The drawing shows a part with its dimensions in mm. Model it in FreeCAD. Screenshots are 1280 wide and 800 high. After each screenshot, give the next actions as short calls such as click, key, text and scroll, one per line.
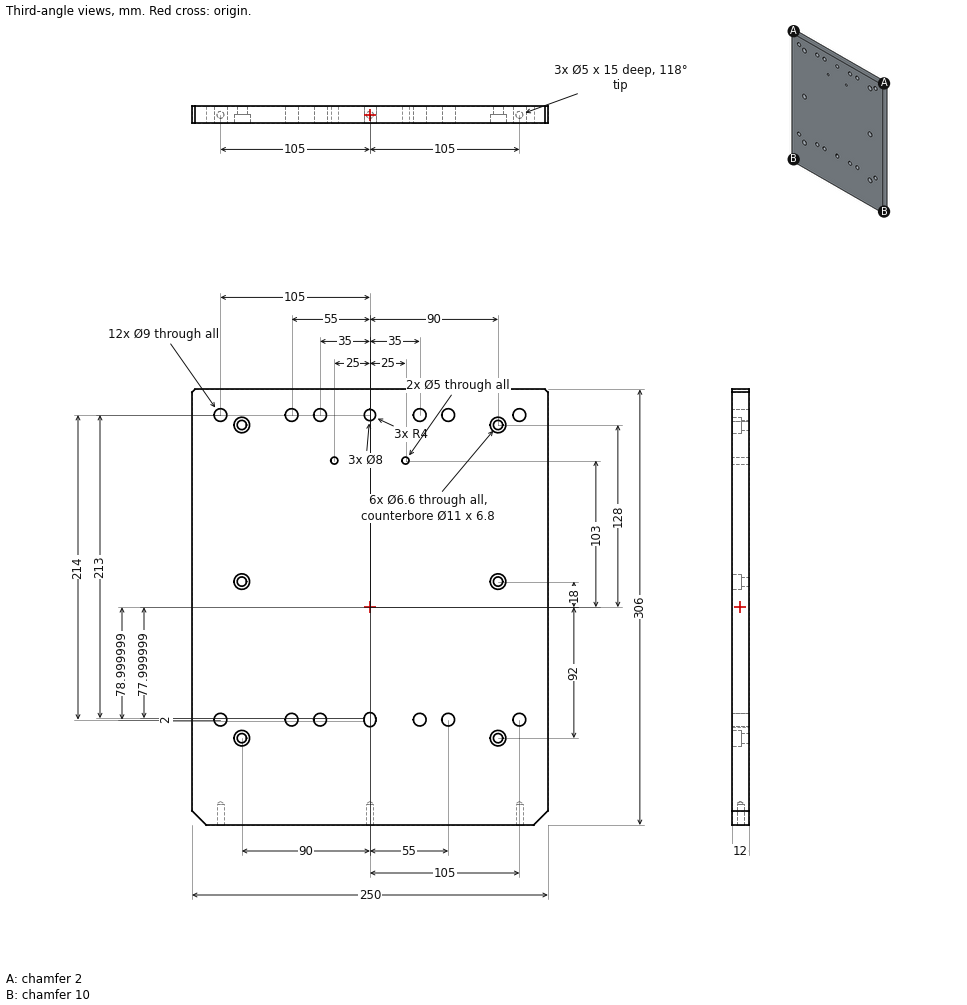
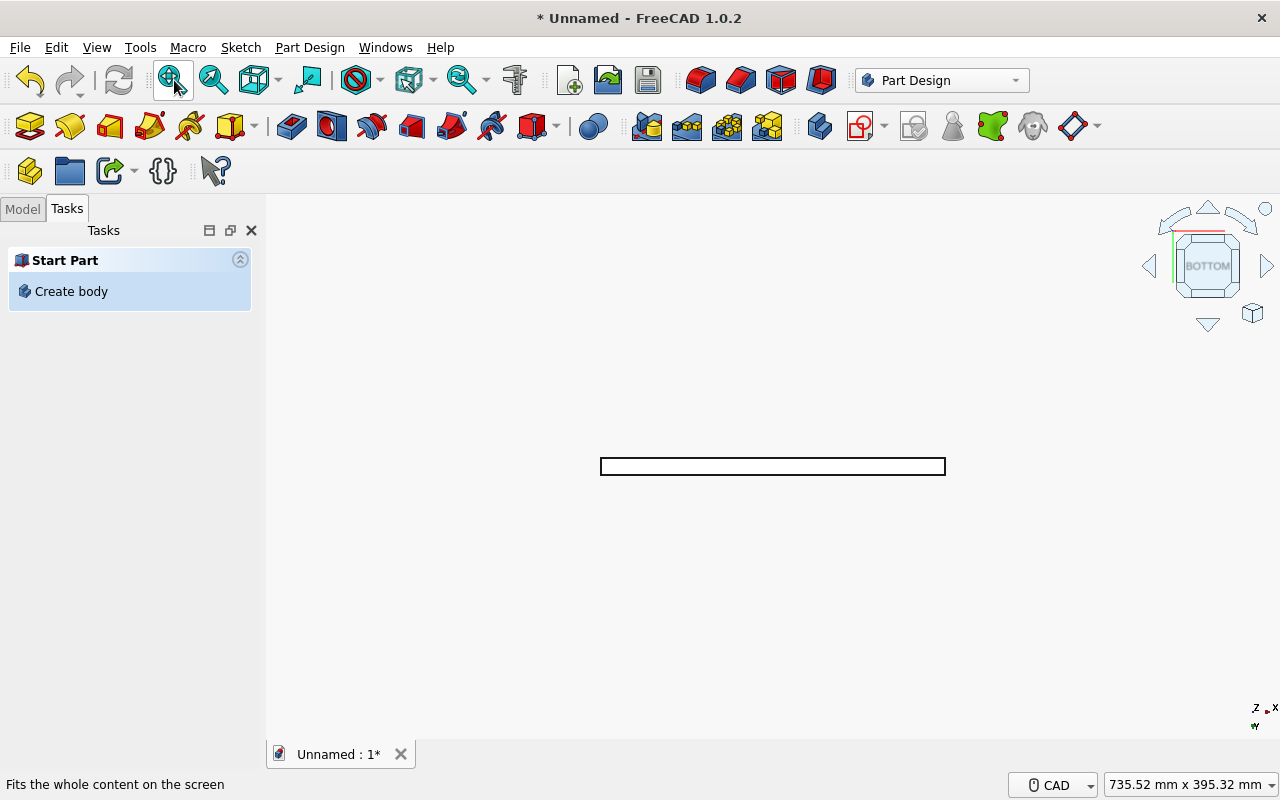
key(1)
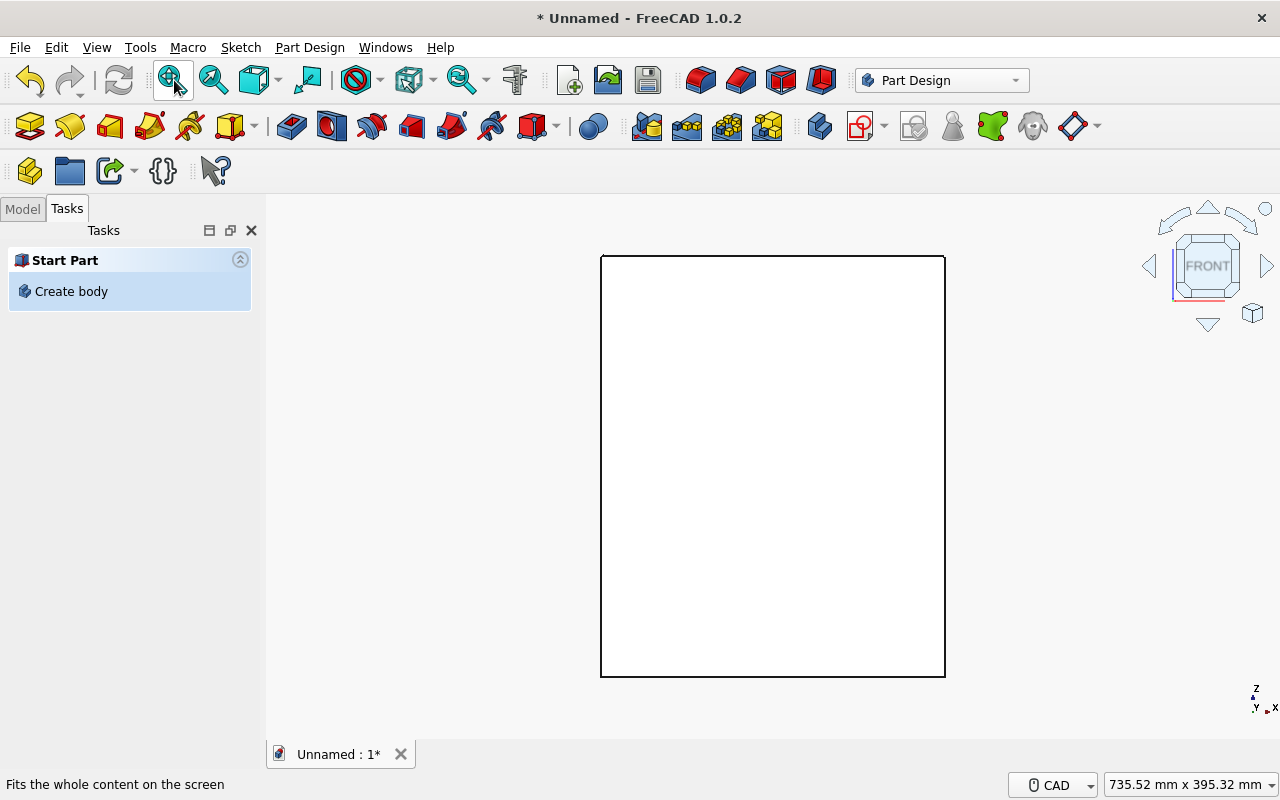
key(3)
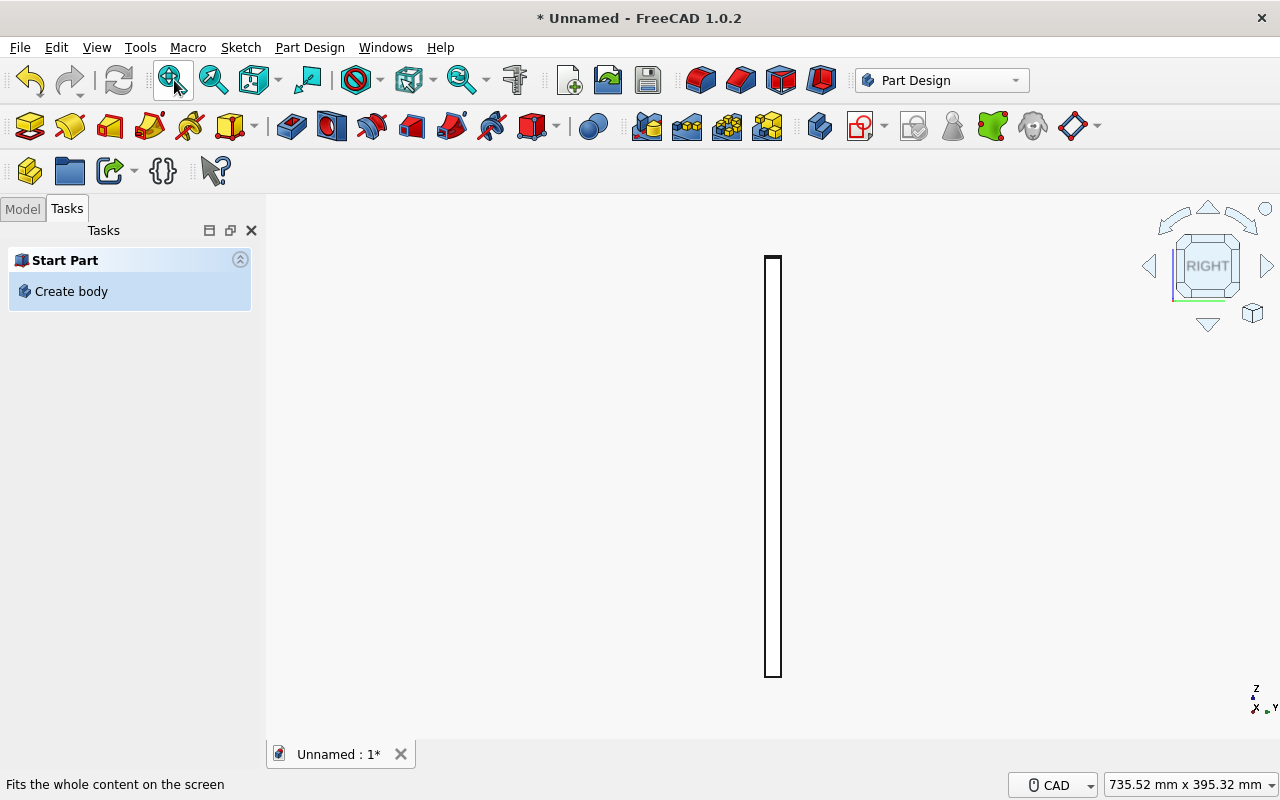
click(23, 208)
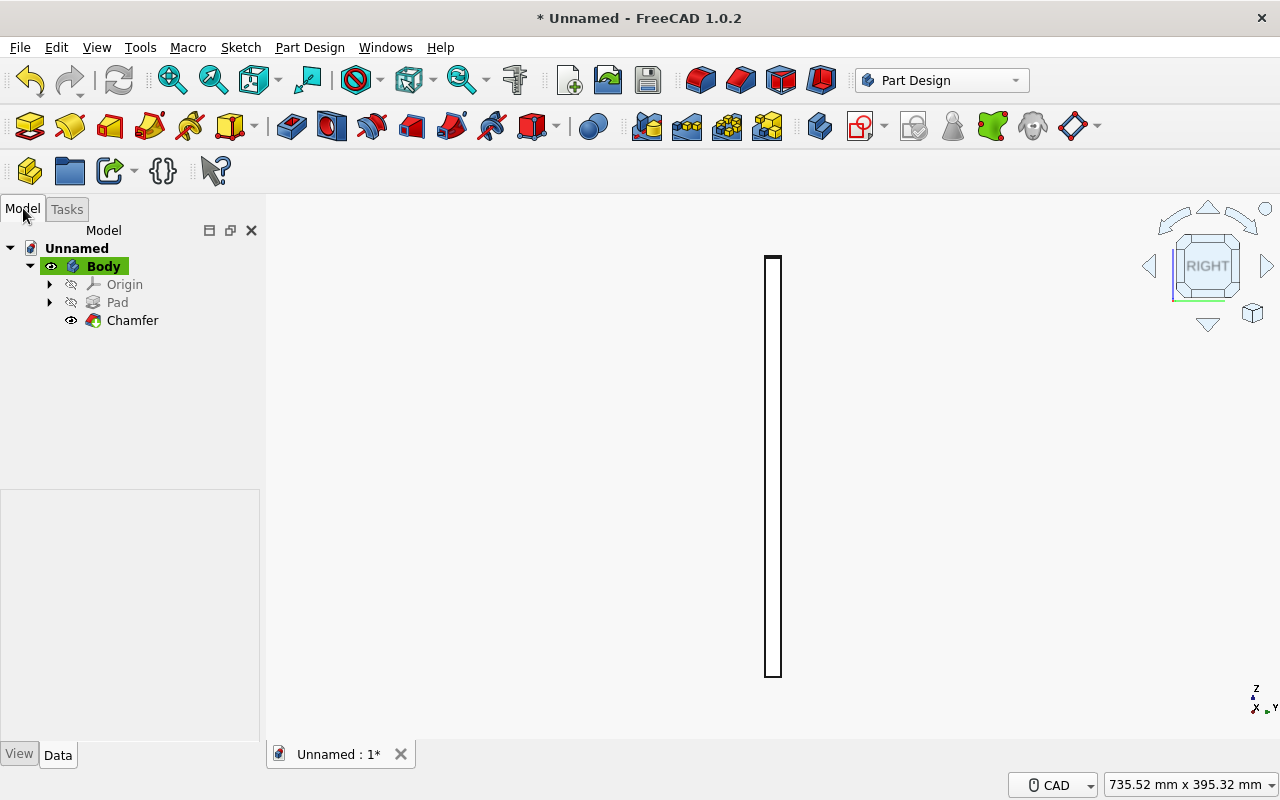
click(50, 284)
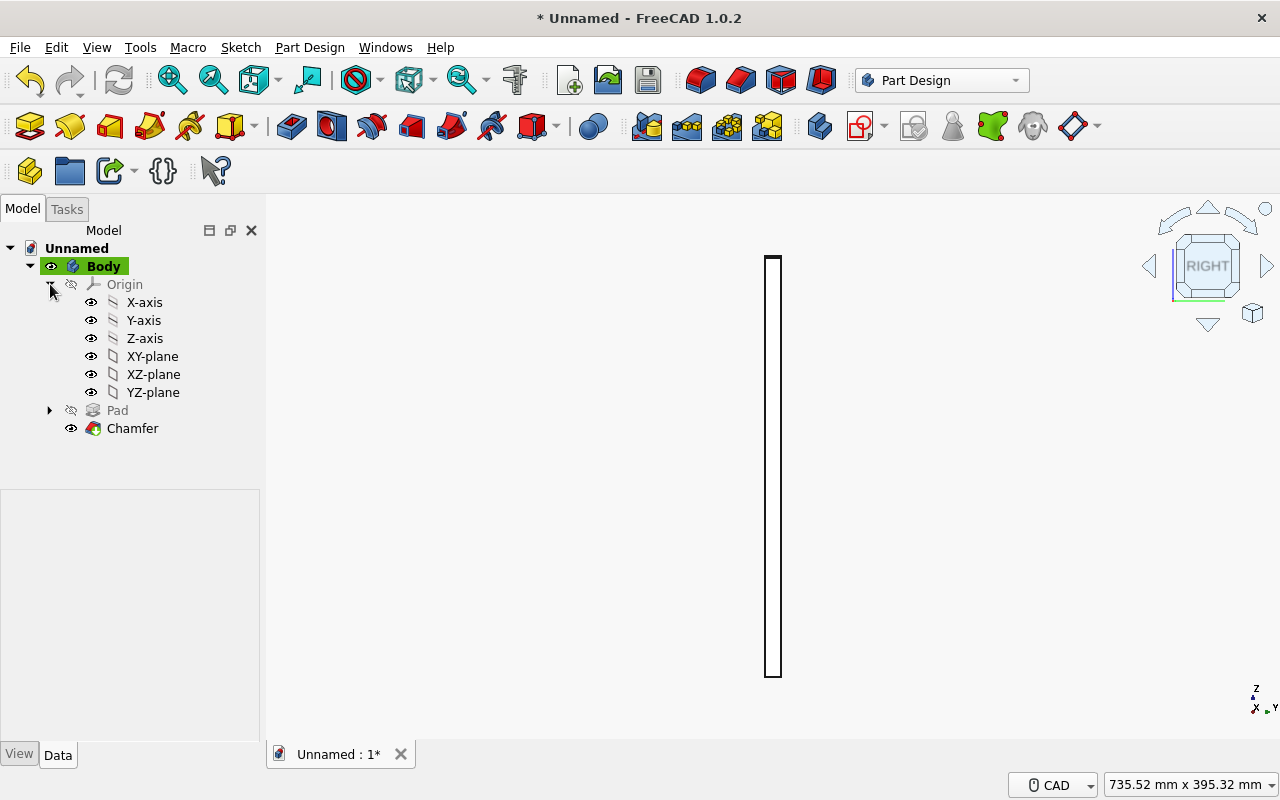
click(136, 356)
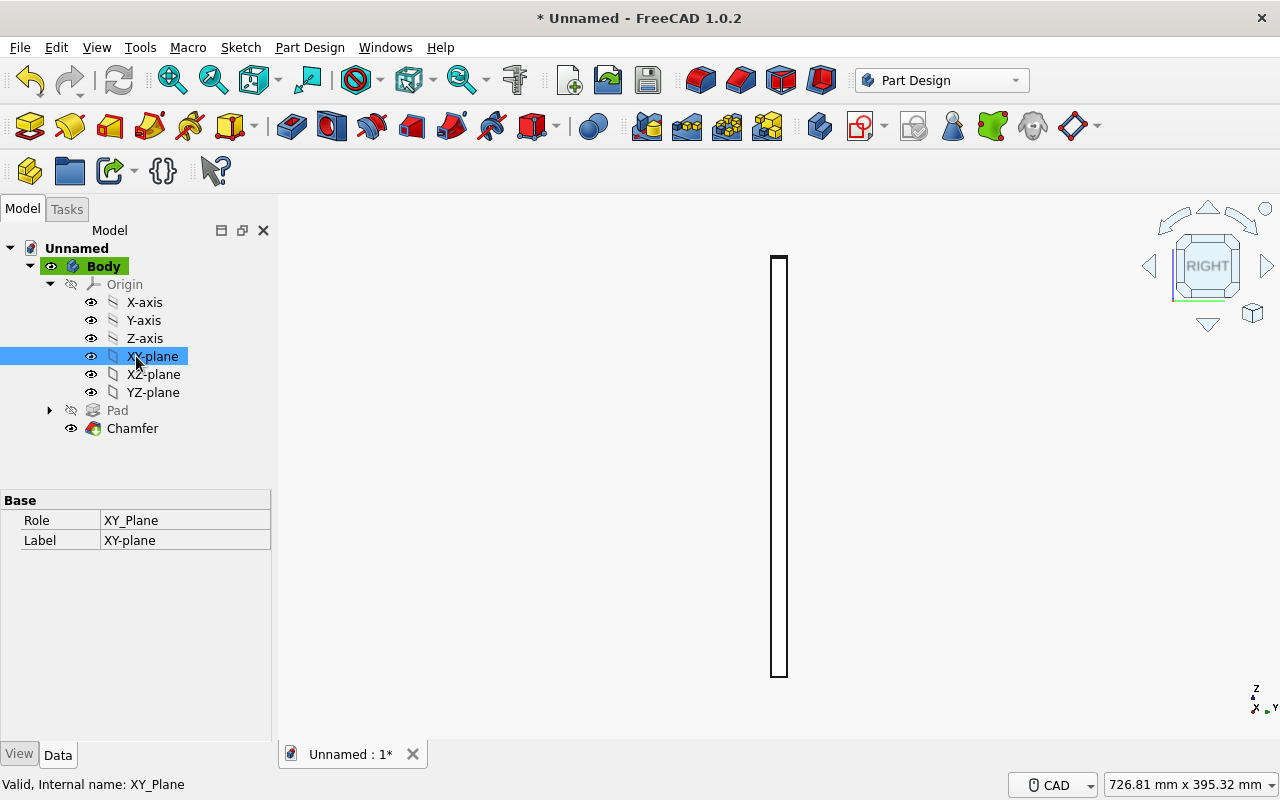
click(1074, 126)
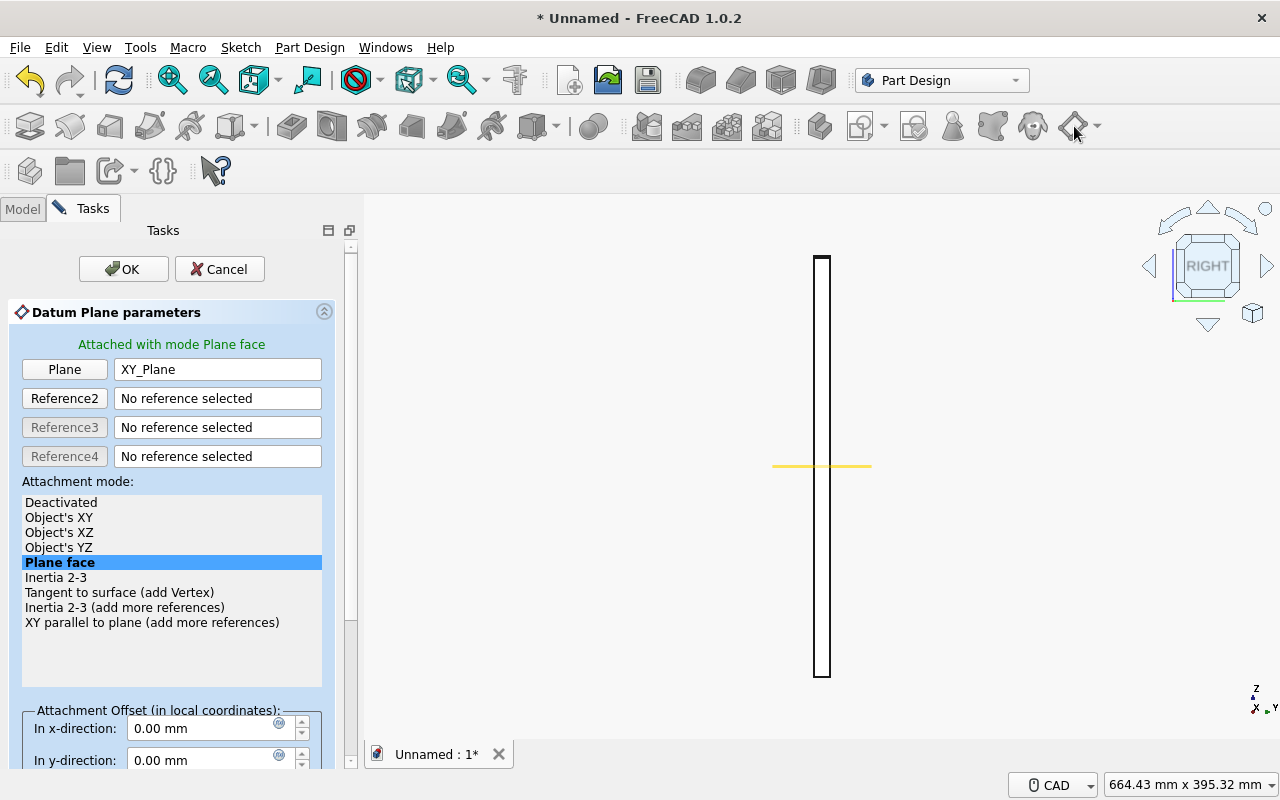
scroll(351, 504, down, 2)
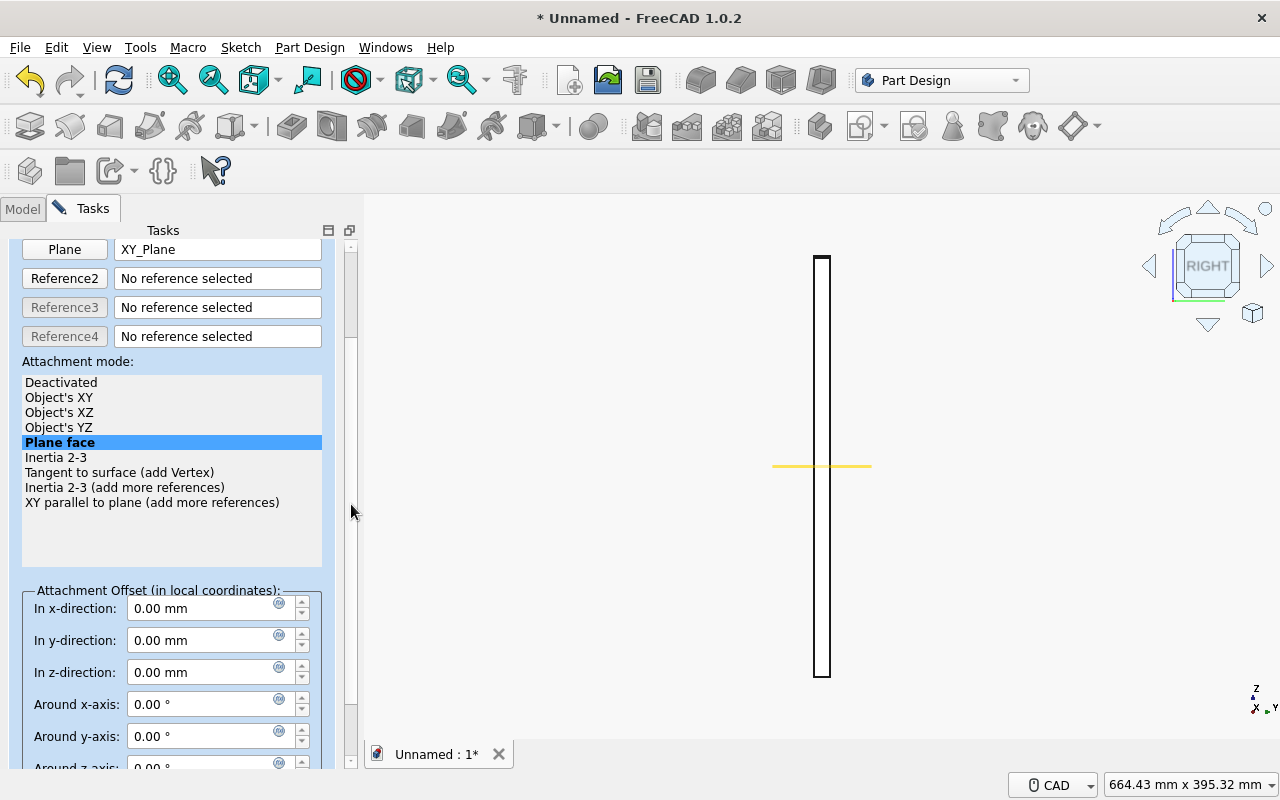
triple_click(210, 672)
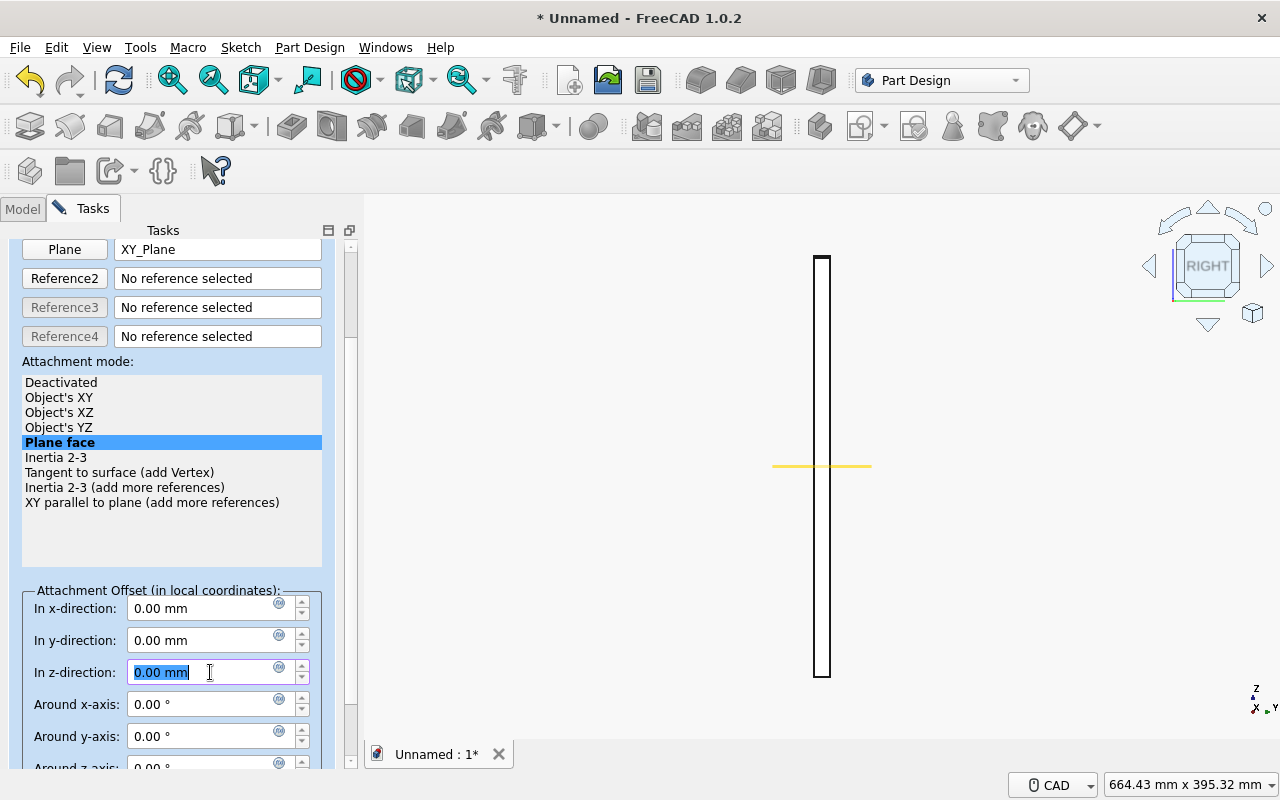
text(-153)
key(Tab)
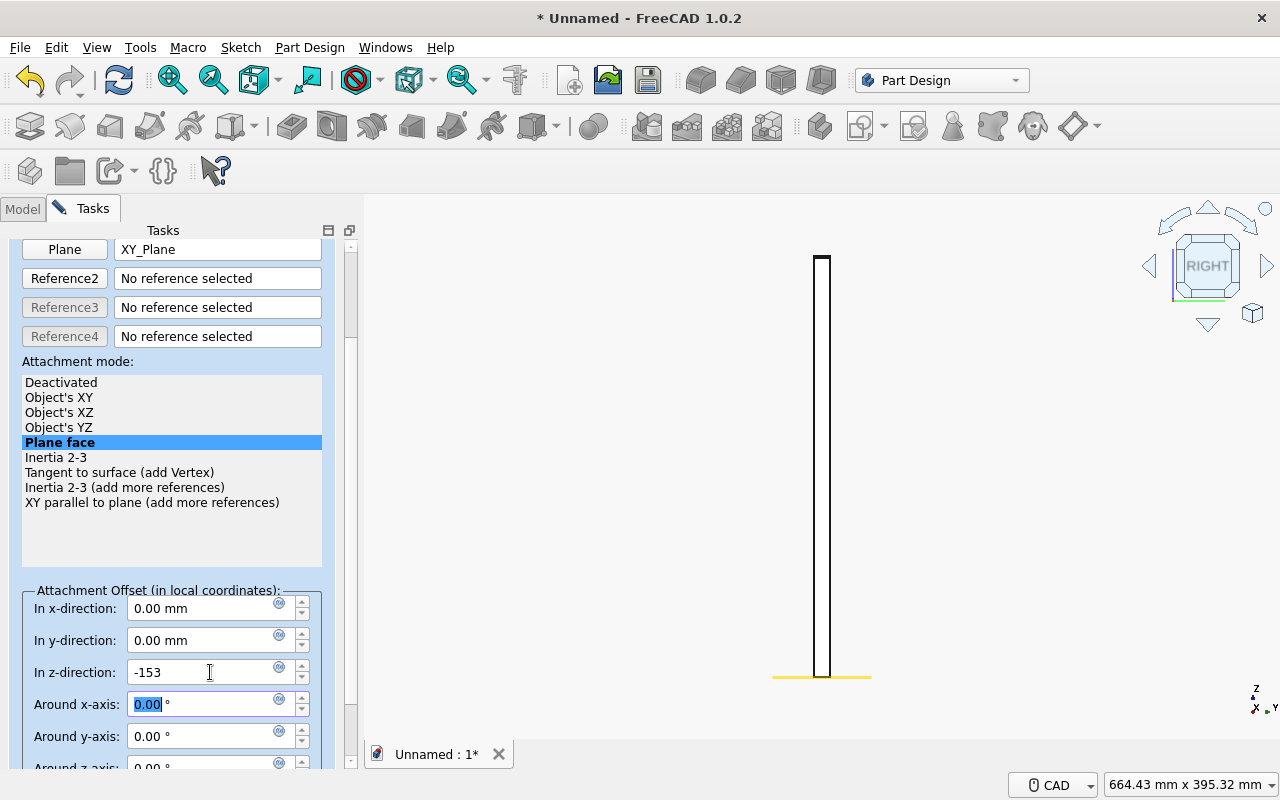
scroll(351, 504, up, 3)